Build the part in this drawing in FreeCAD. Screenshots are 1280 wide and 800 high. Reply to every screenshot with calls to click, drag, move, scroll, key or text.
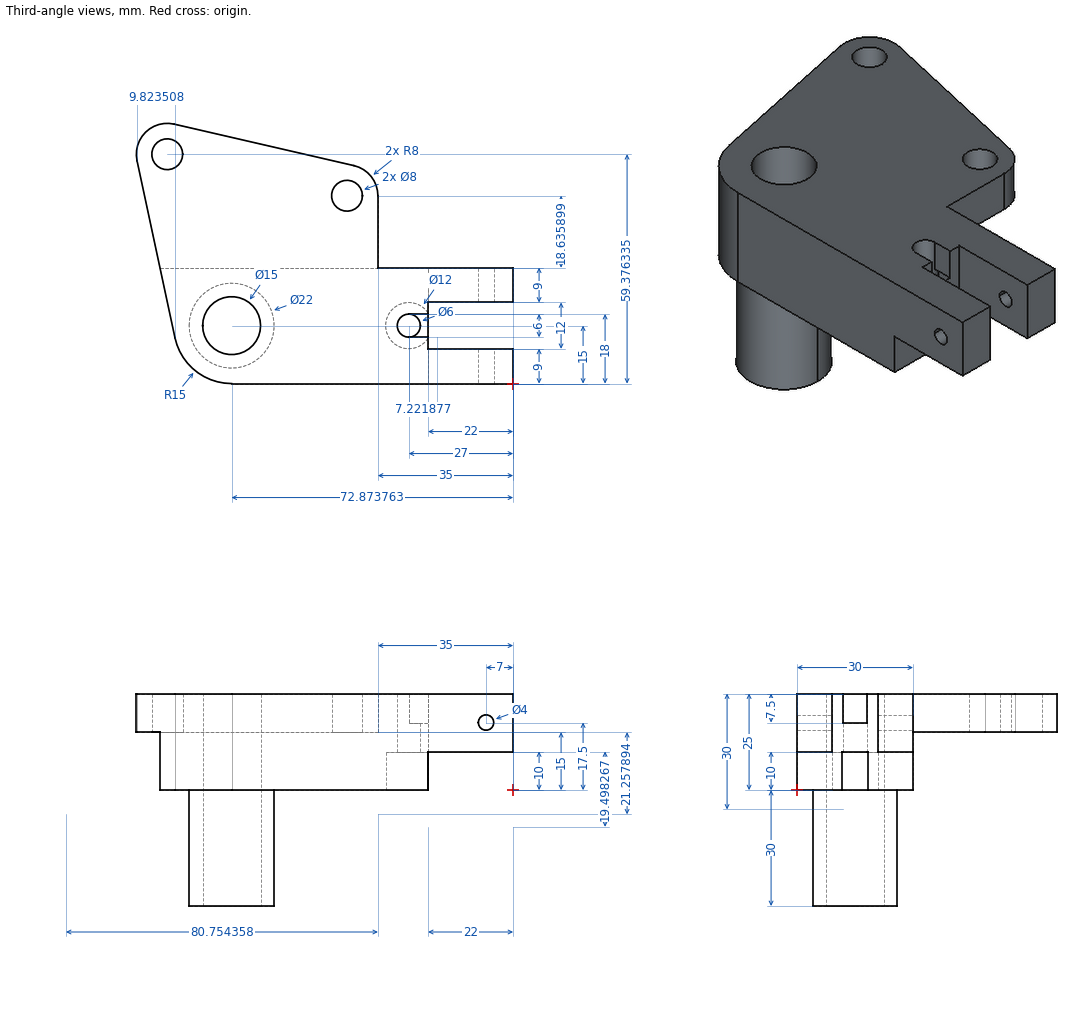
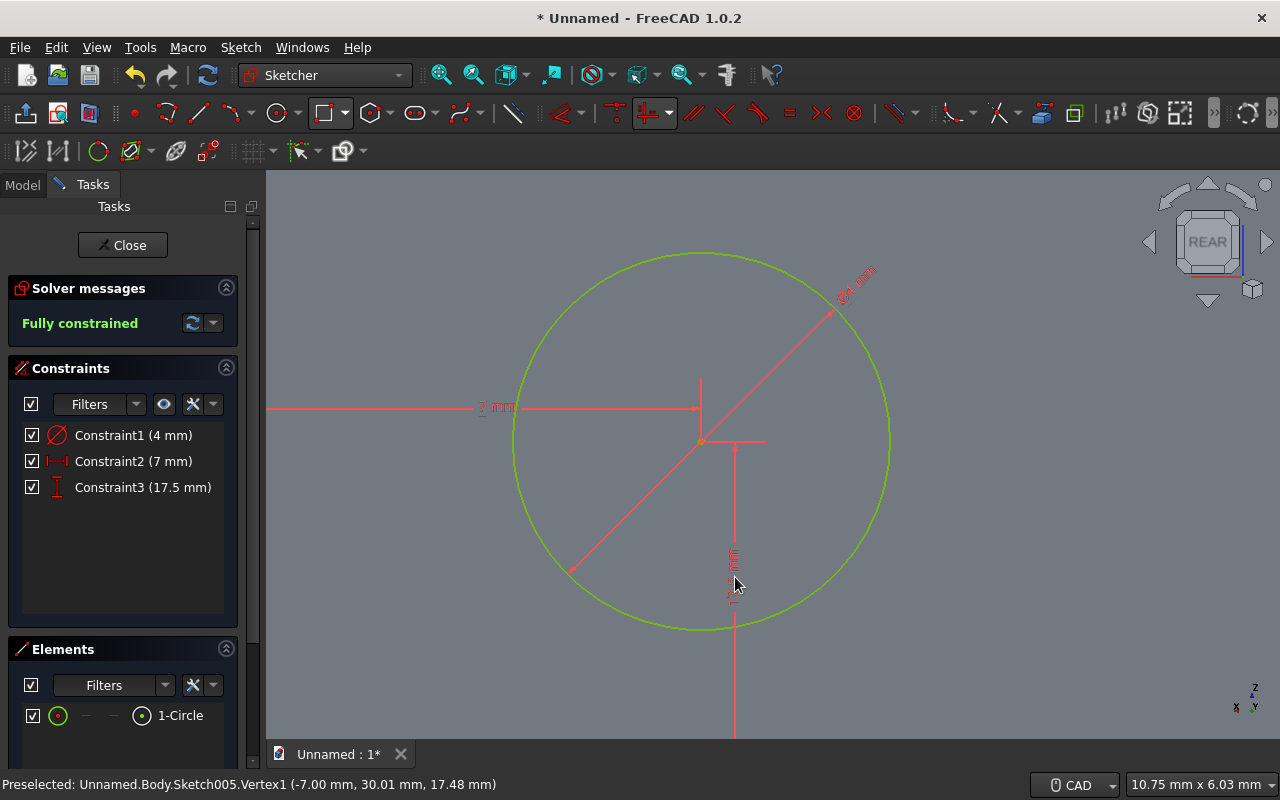
click(123, 245)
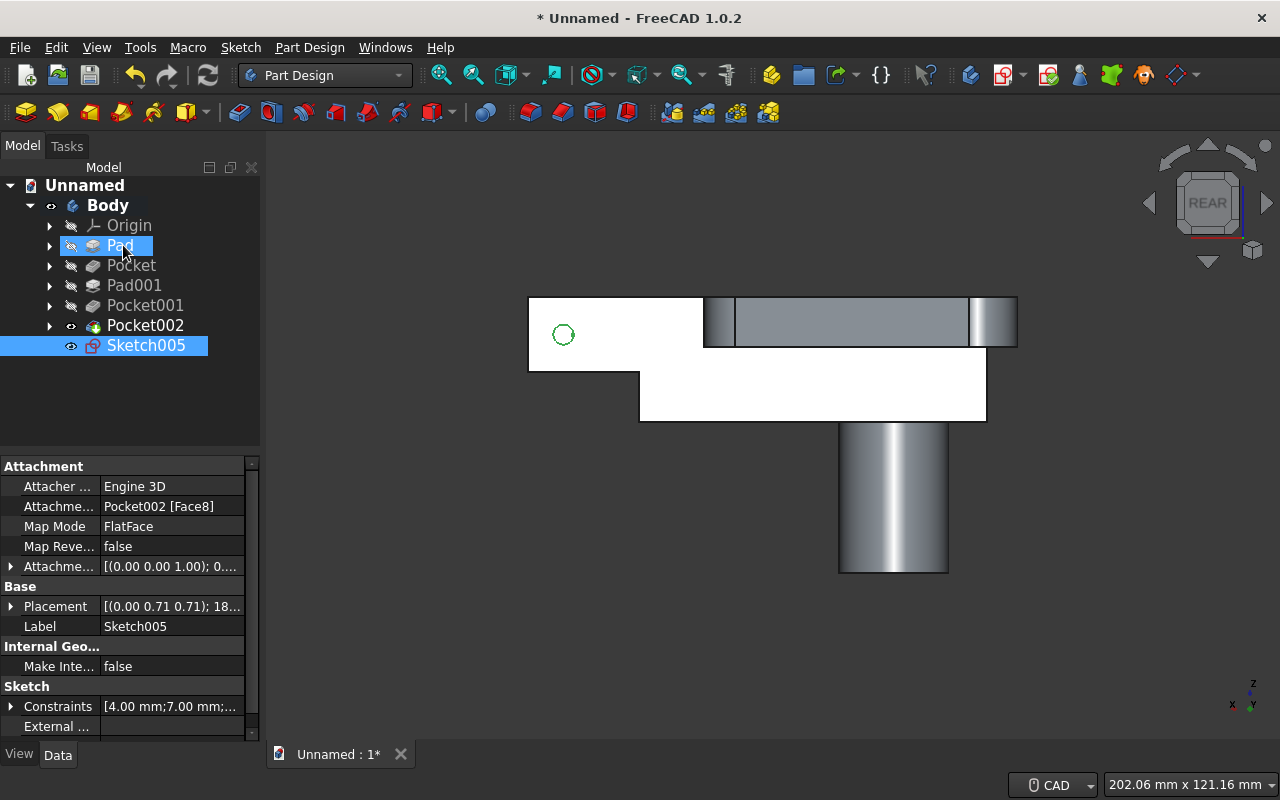
click(240, 112)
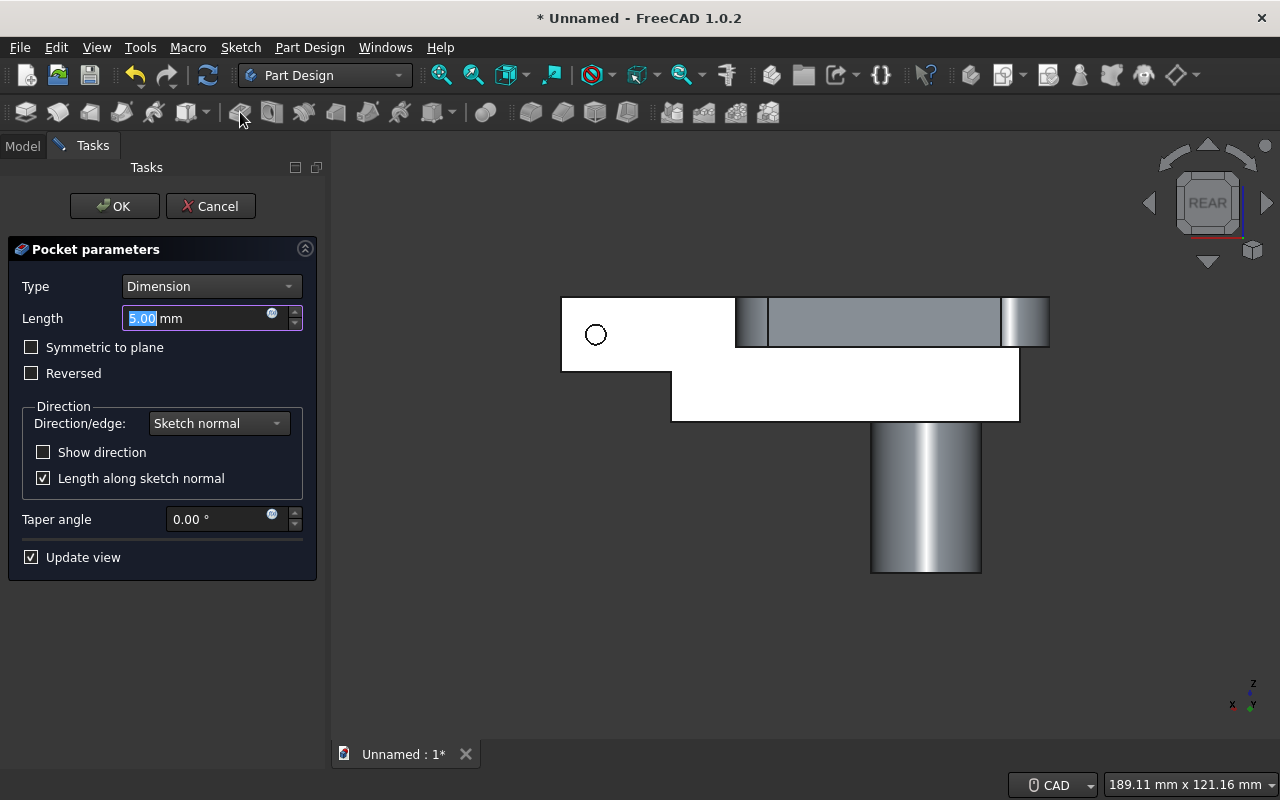
text(30)
key(Tab)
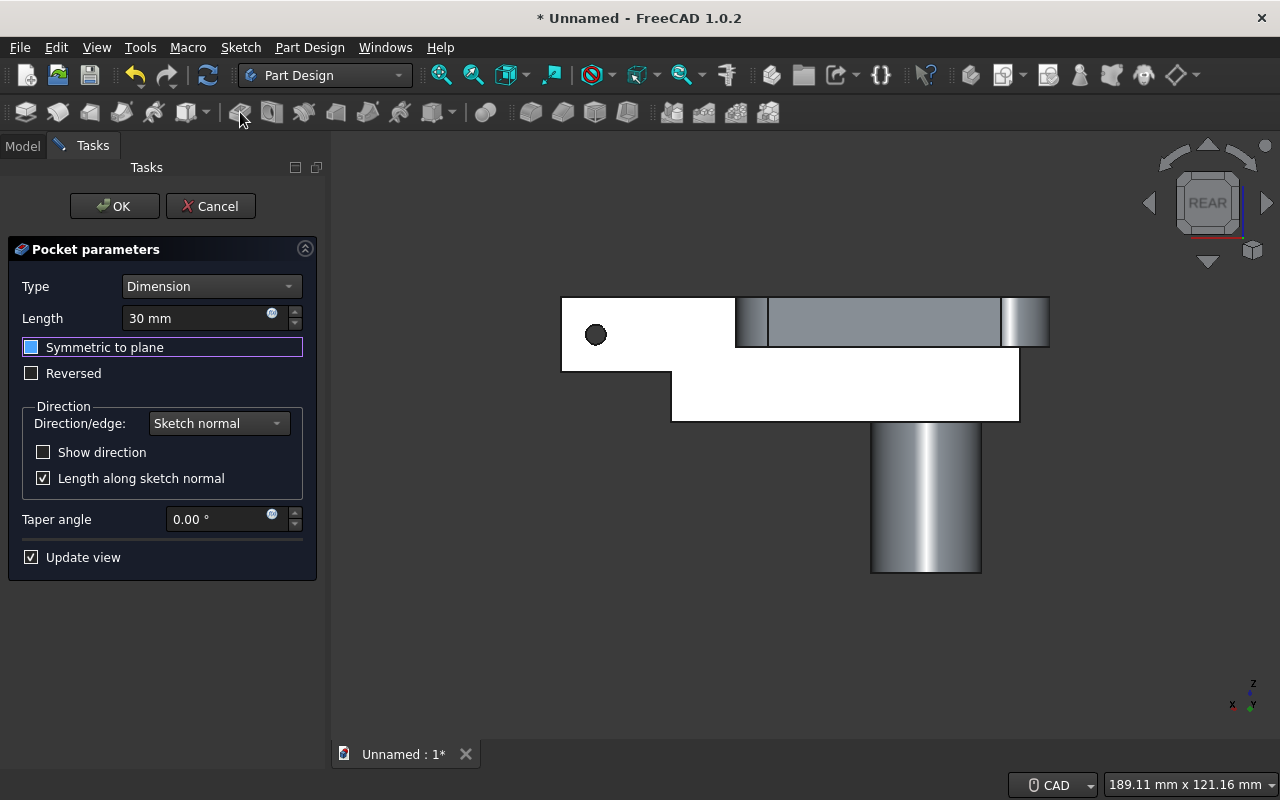
click(115, 206)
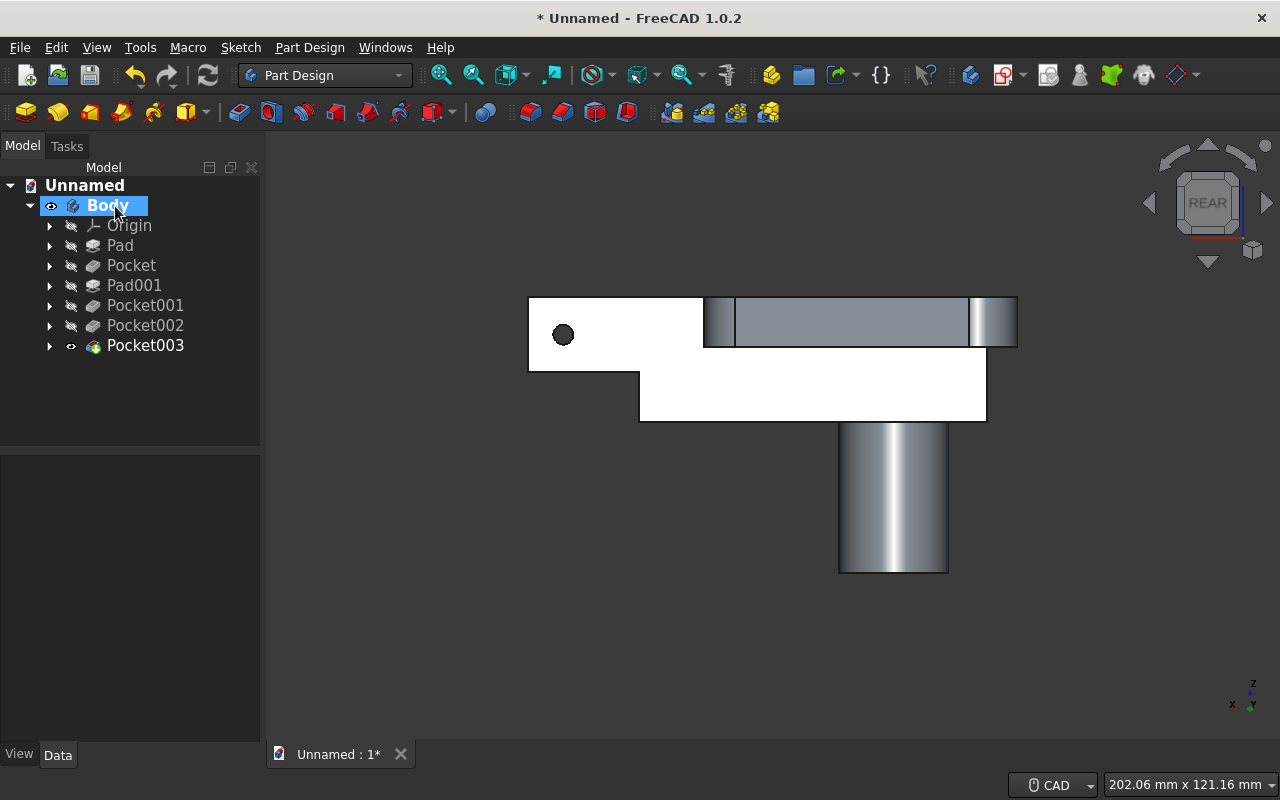
key(0)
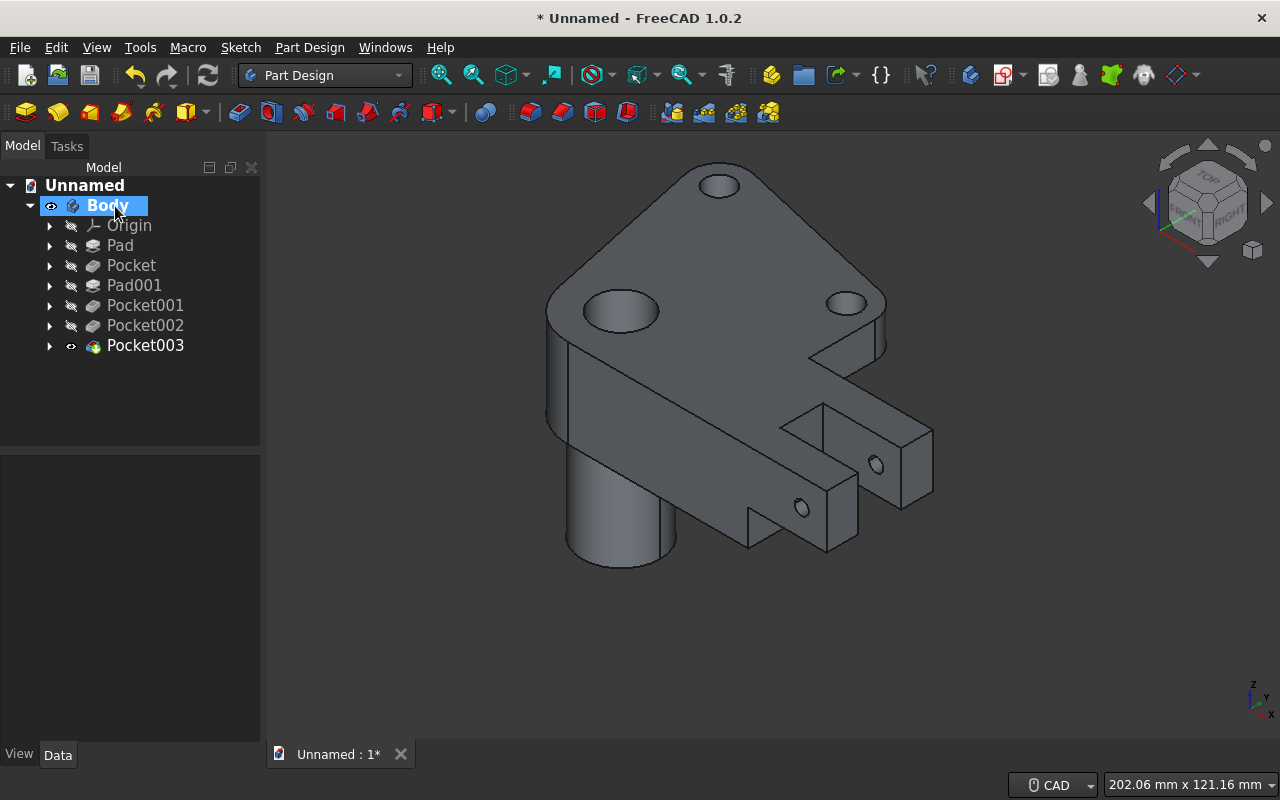
click(708, 245)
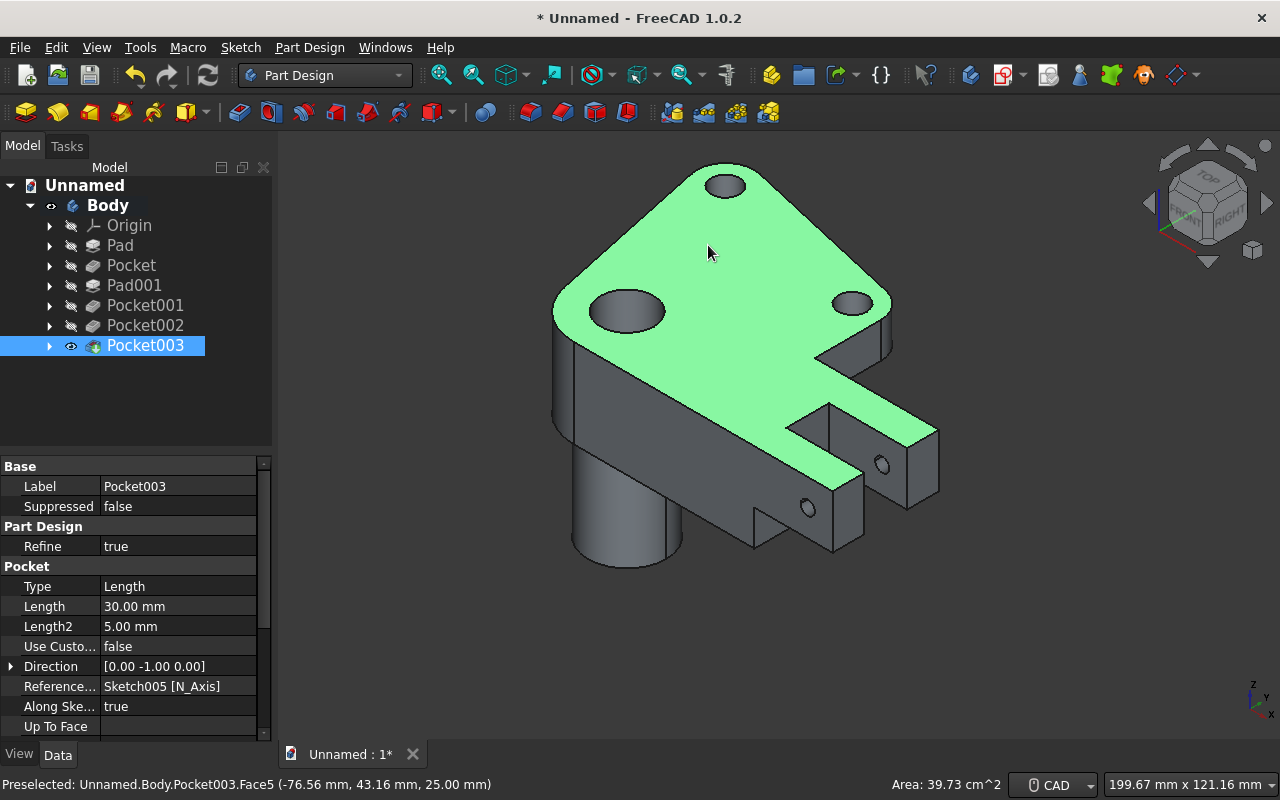
click(1004, 76)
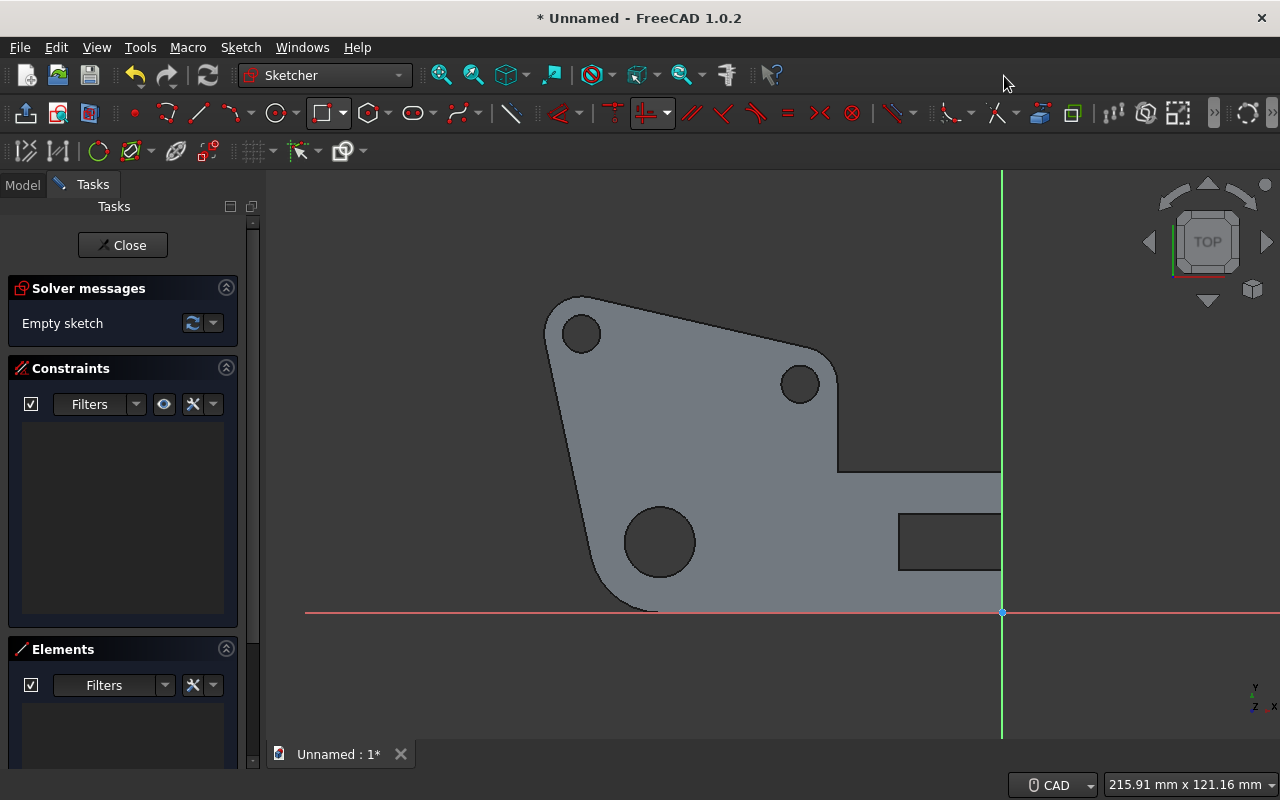
scroll(889, 549, up, 13)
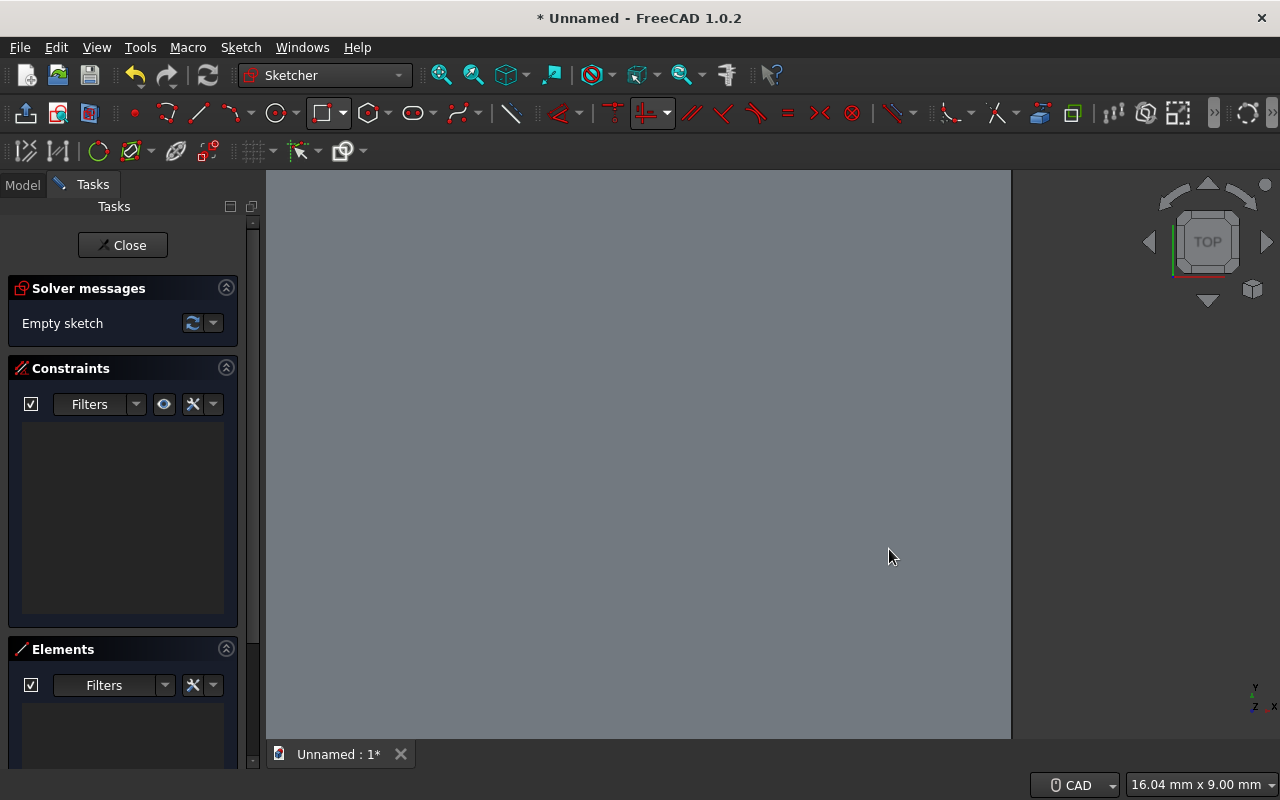
click(276, 114)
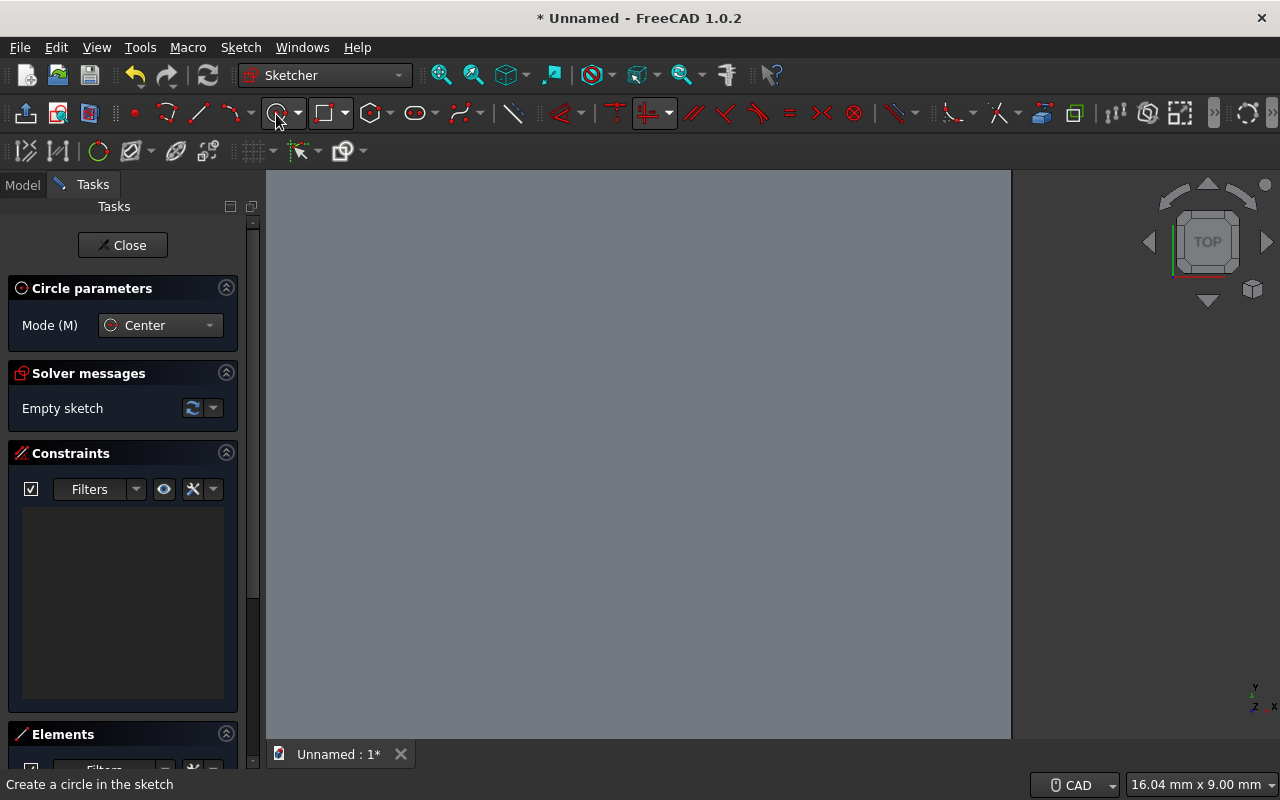
click(696, 450)
click(830, 316)
key(Escape)